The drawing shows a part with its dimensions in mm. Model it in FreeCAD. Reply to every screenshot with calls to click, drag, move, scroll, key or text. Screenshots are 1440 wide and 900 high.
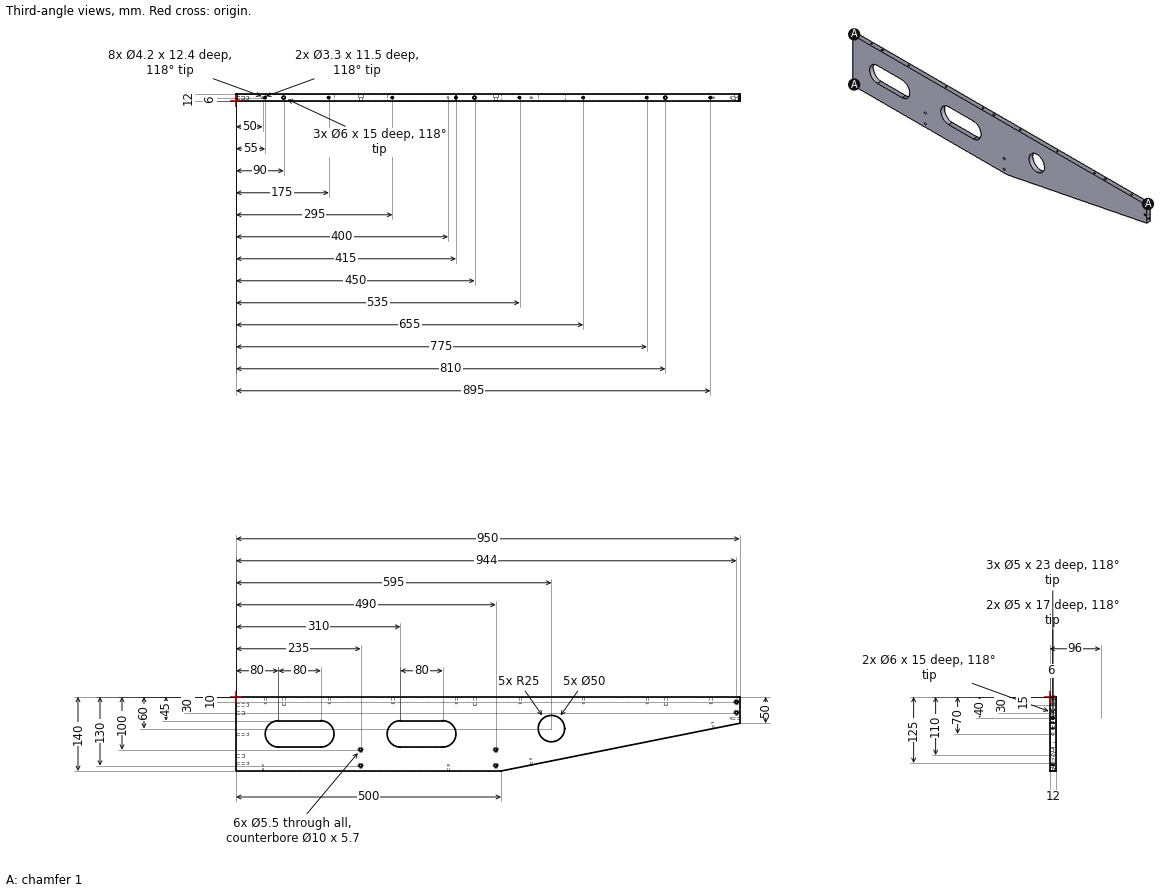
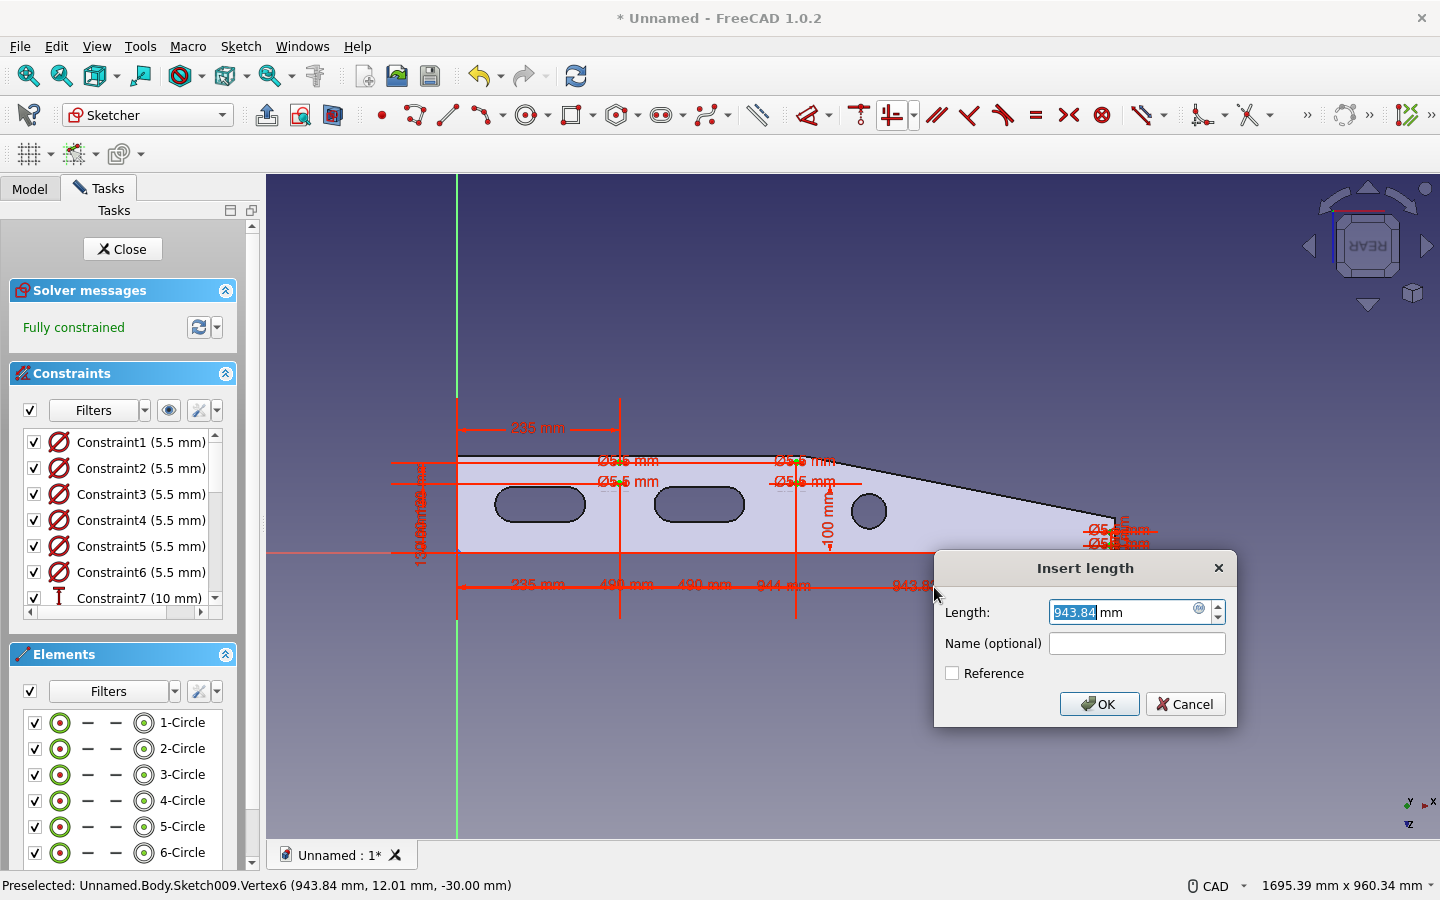
text(944)
key(Return)
key(Escape)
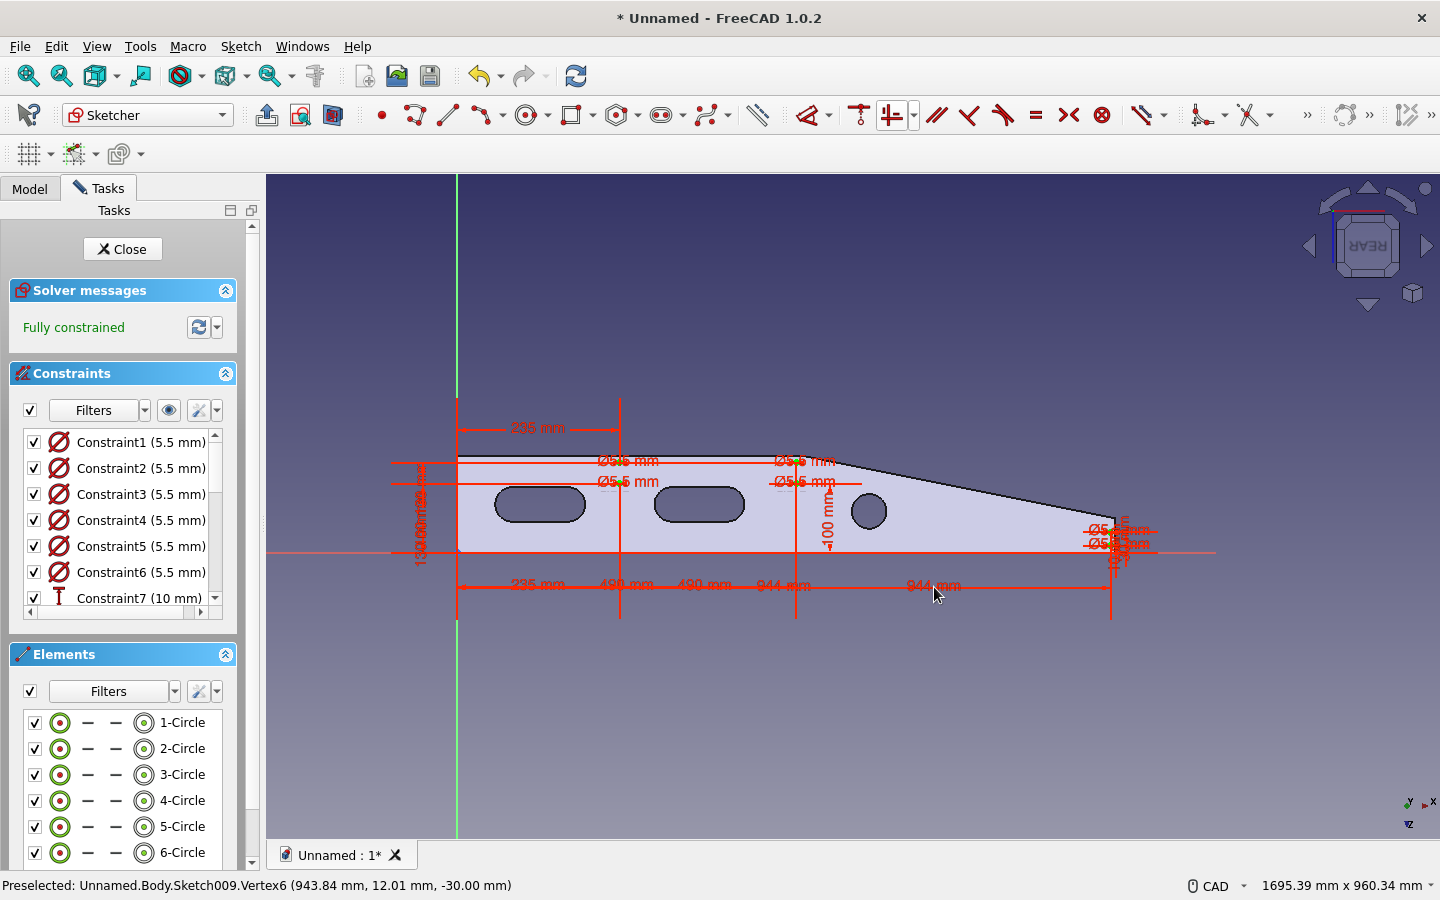
click(123, 249)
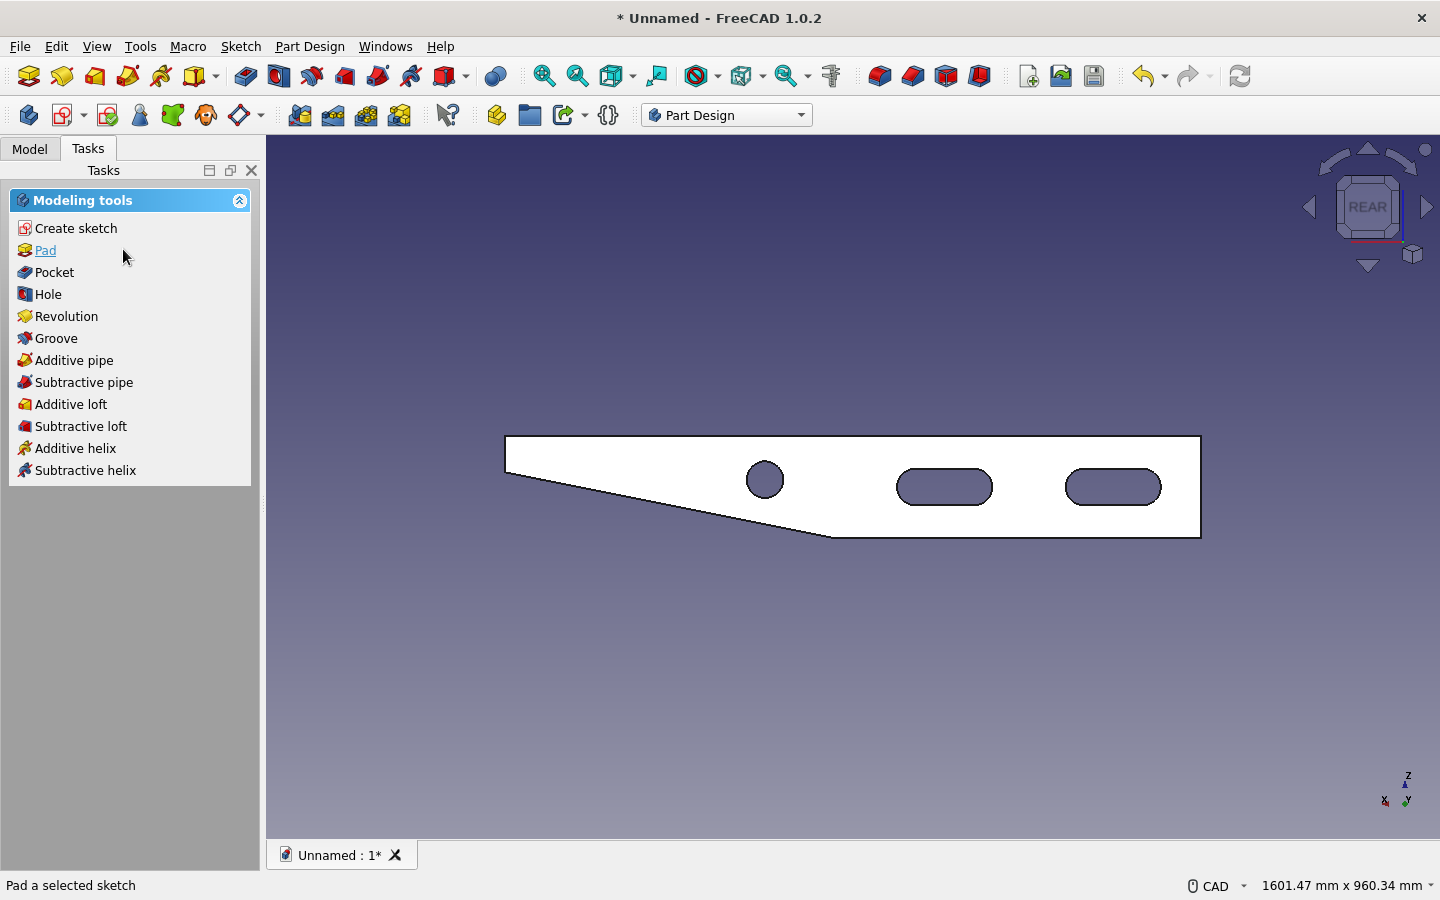
click(279, 76)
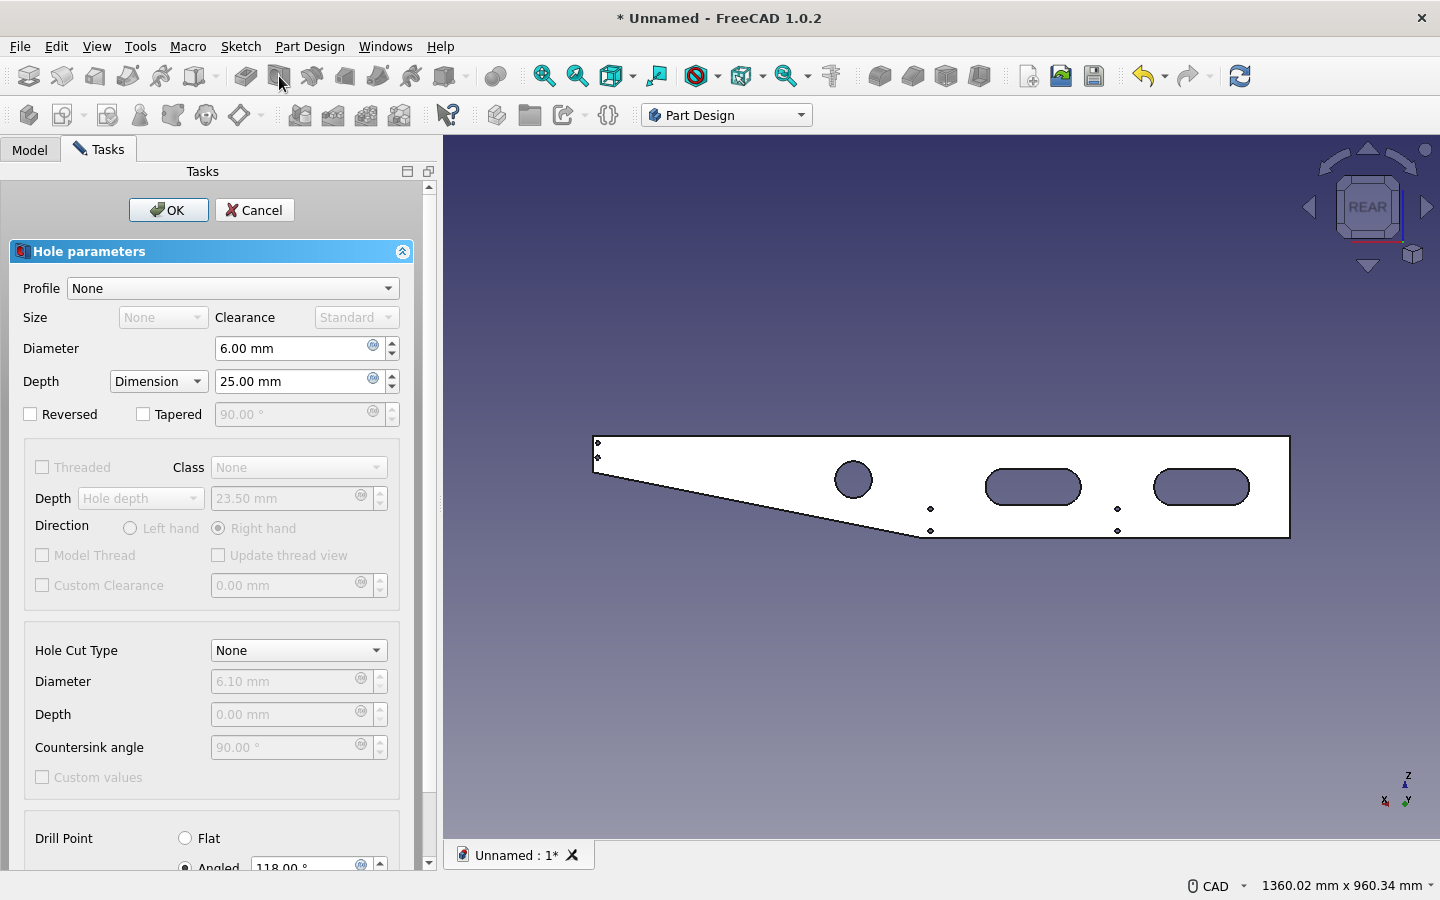
triple_click(300, 348)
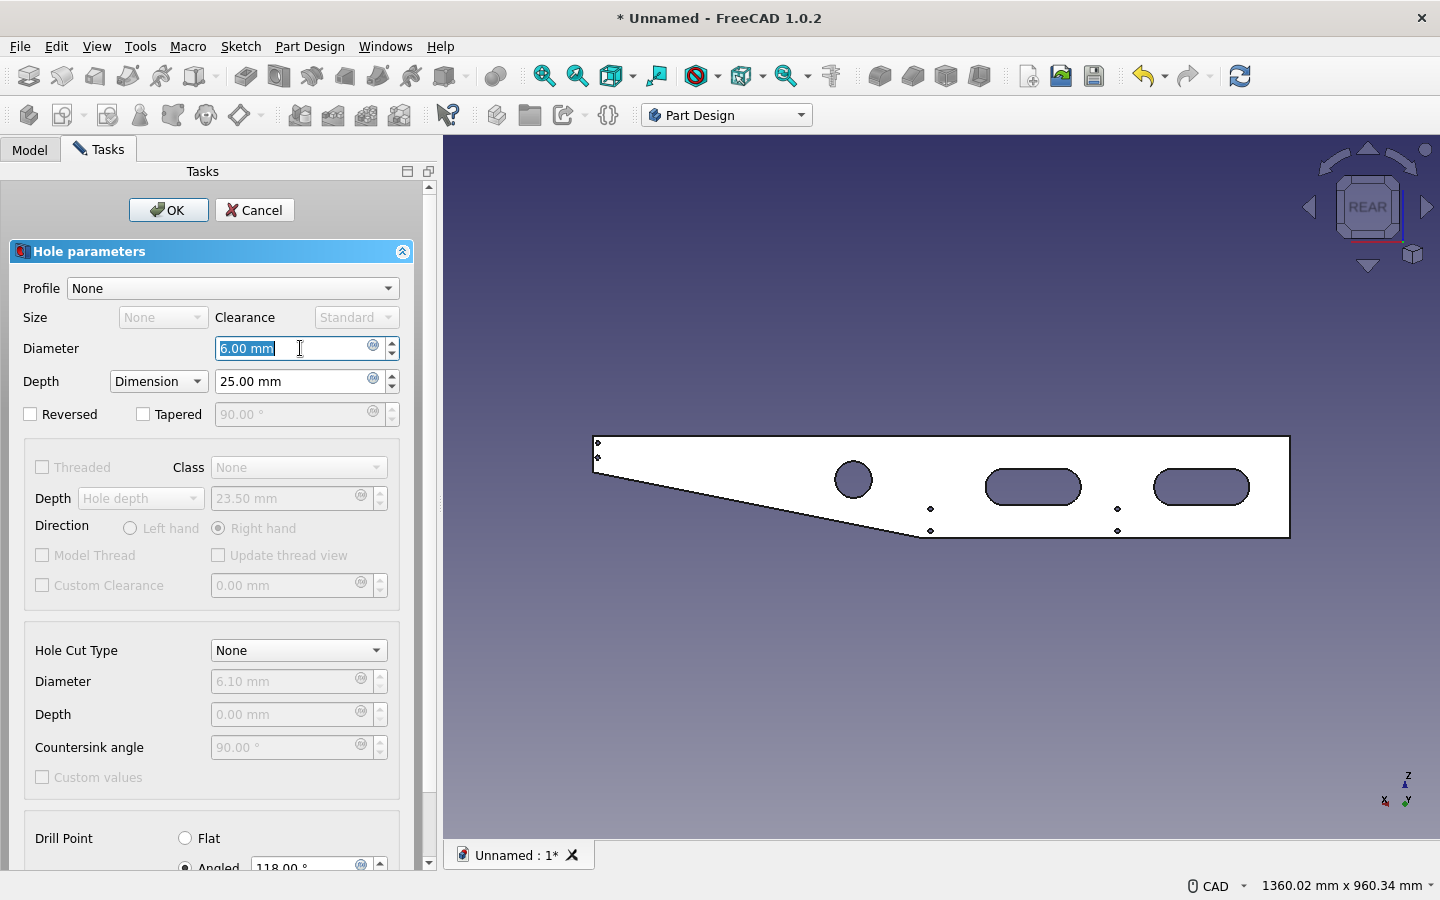
text(5.5)
key(Tab)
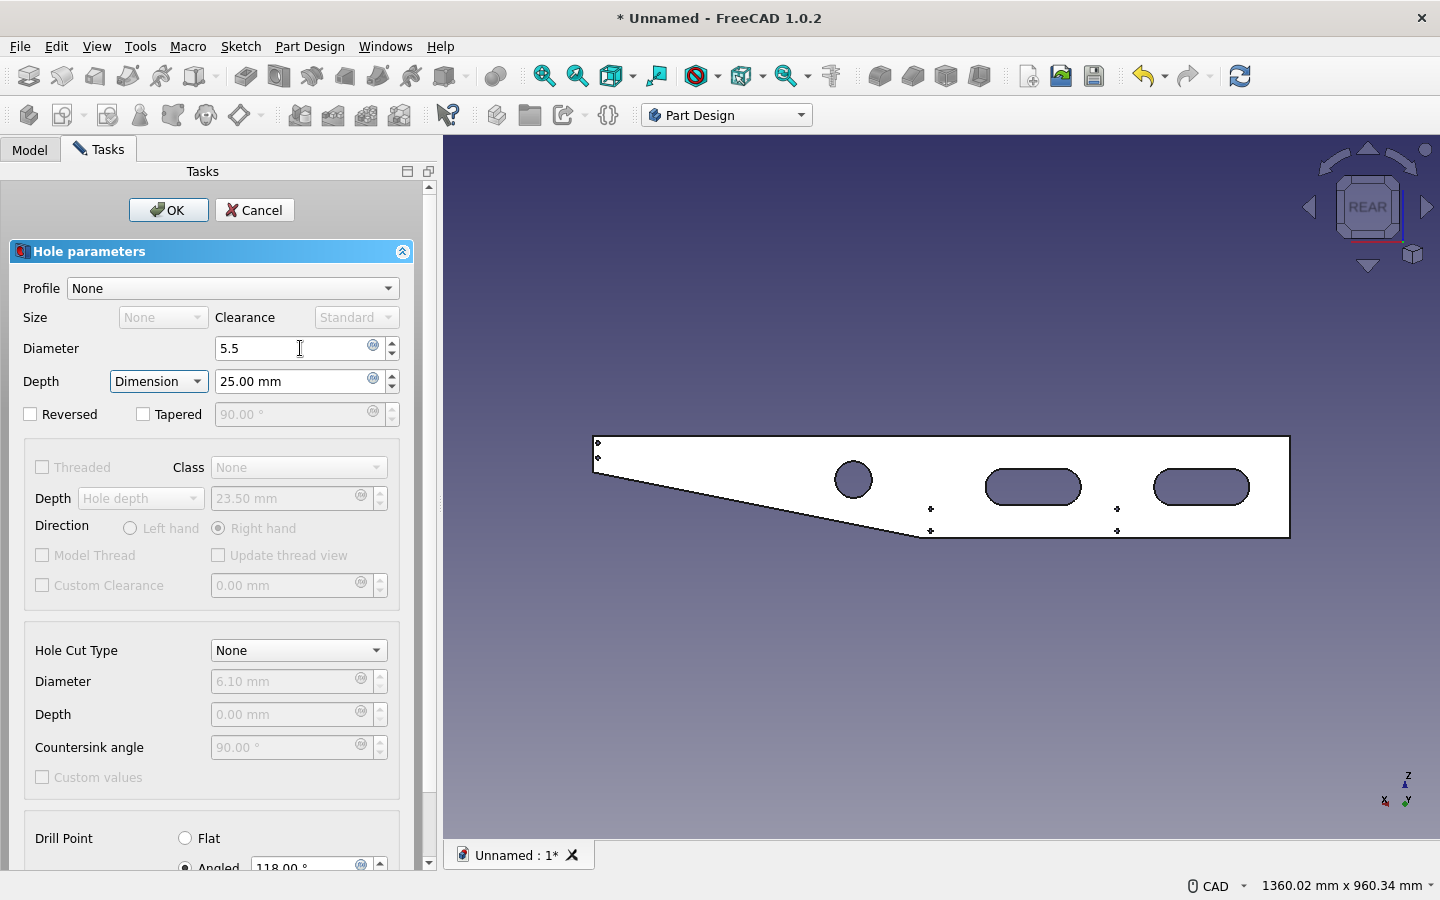
click(160, 382)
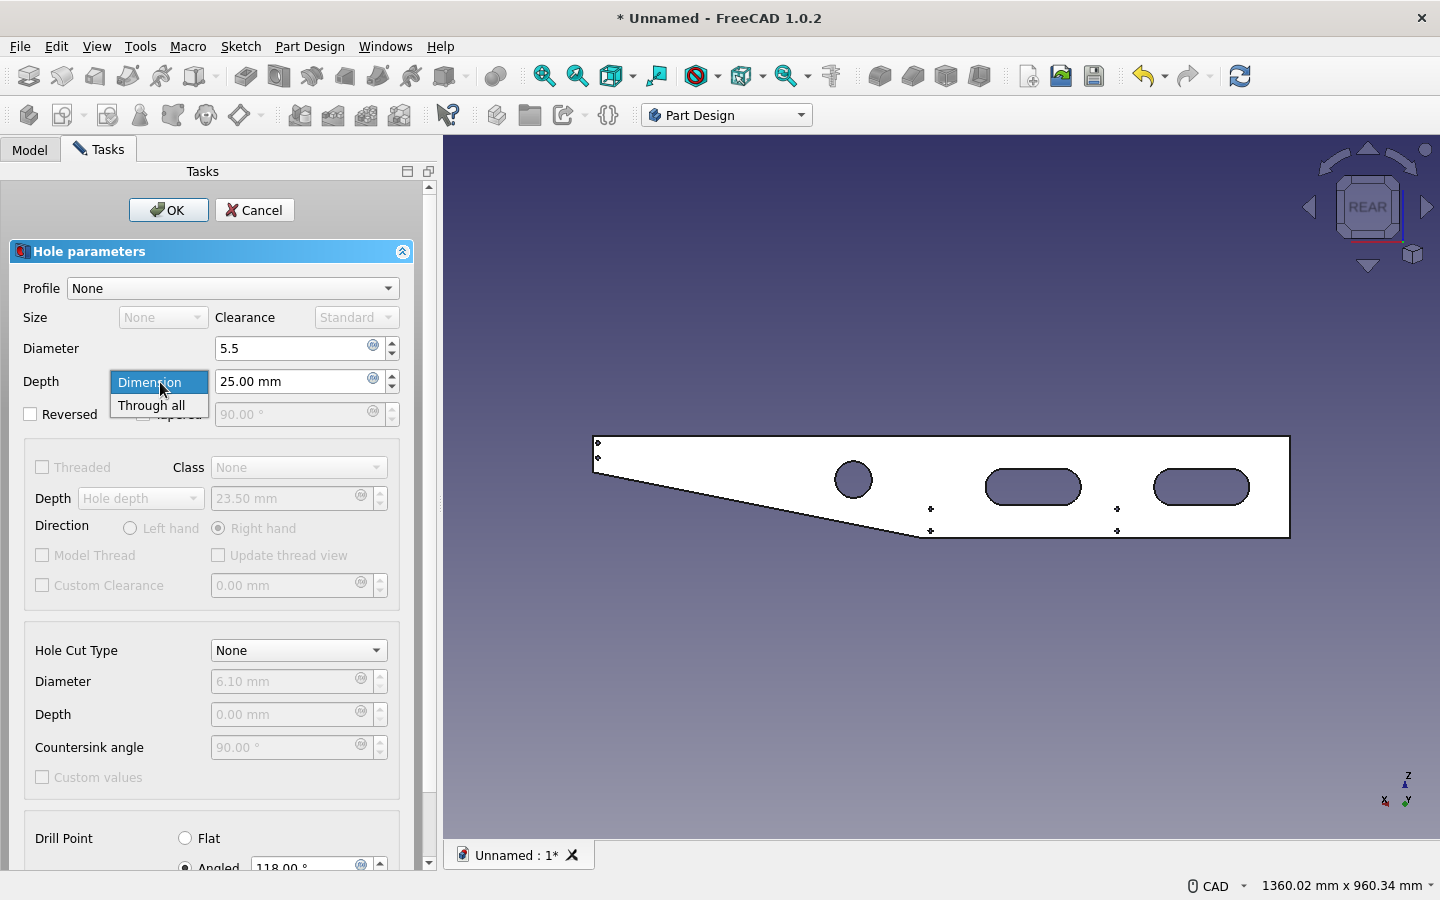
click(158, 406)